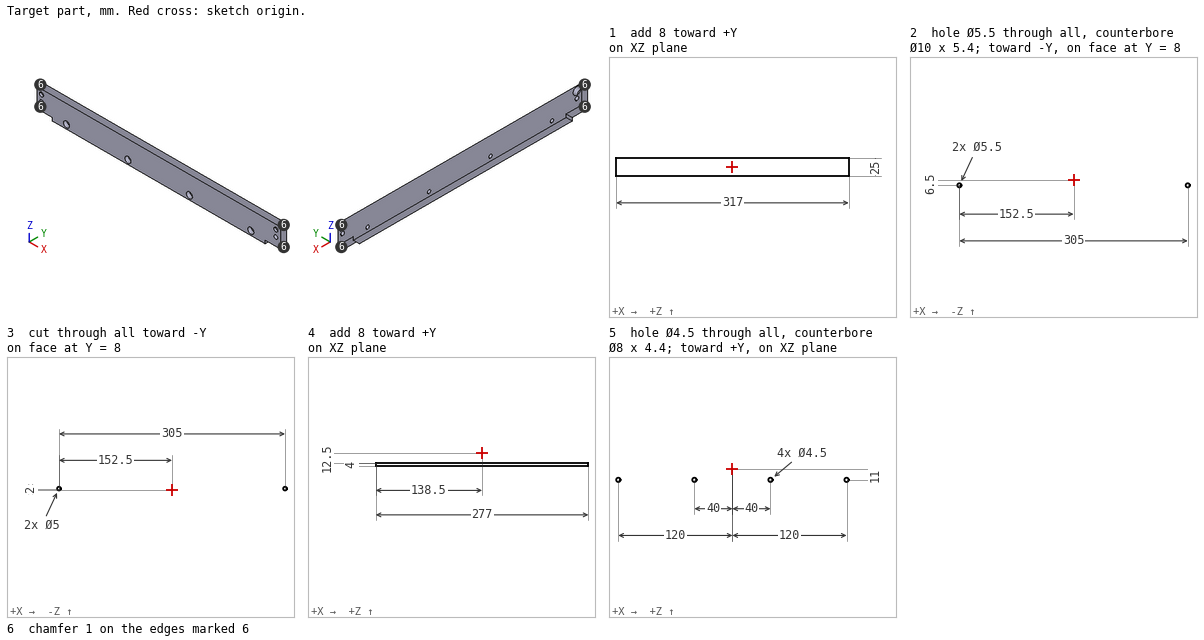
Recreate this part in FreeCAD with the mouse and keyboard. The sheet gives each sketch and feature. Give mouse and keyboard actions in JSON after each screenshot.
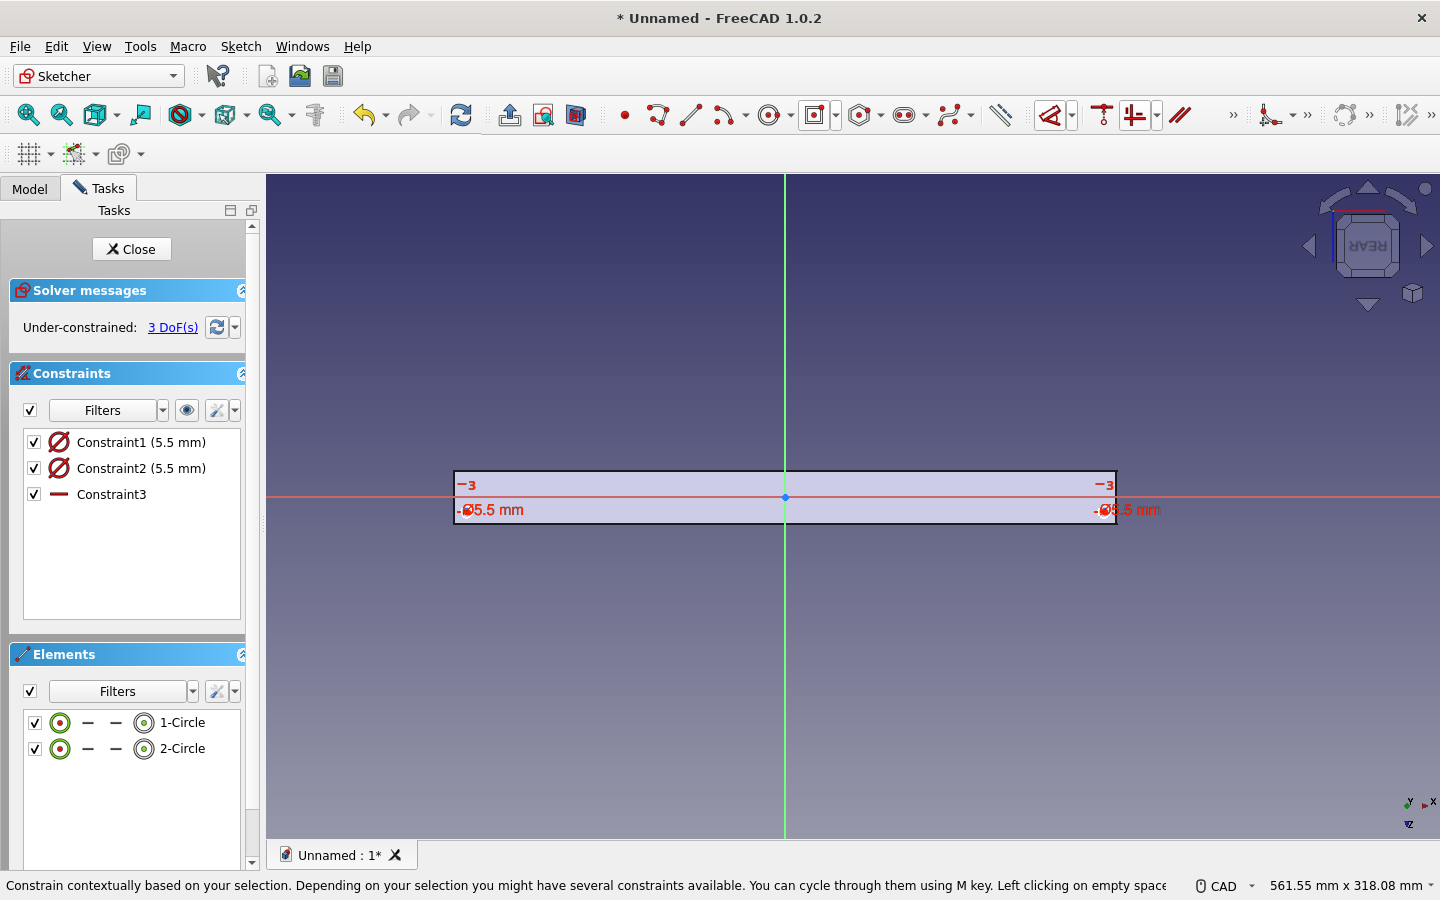
{"action": "scroll", "coordinate": [467, 512], "scroll_direction": "up", "scroll_amount": 6}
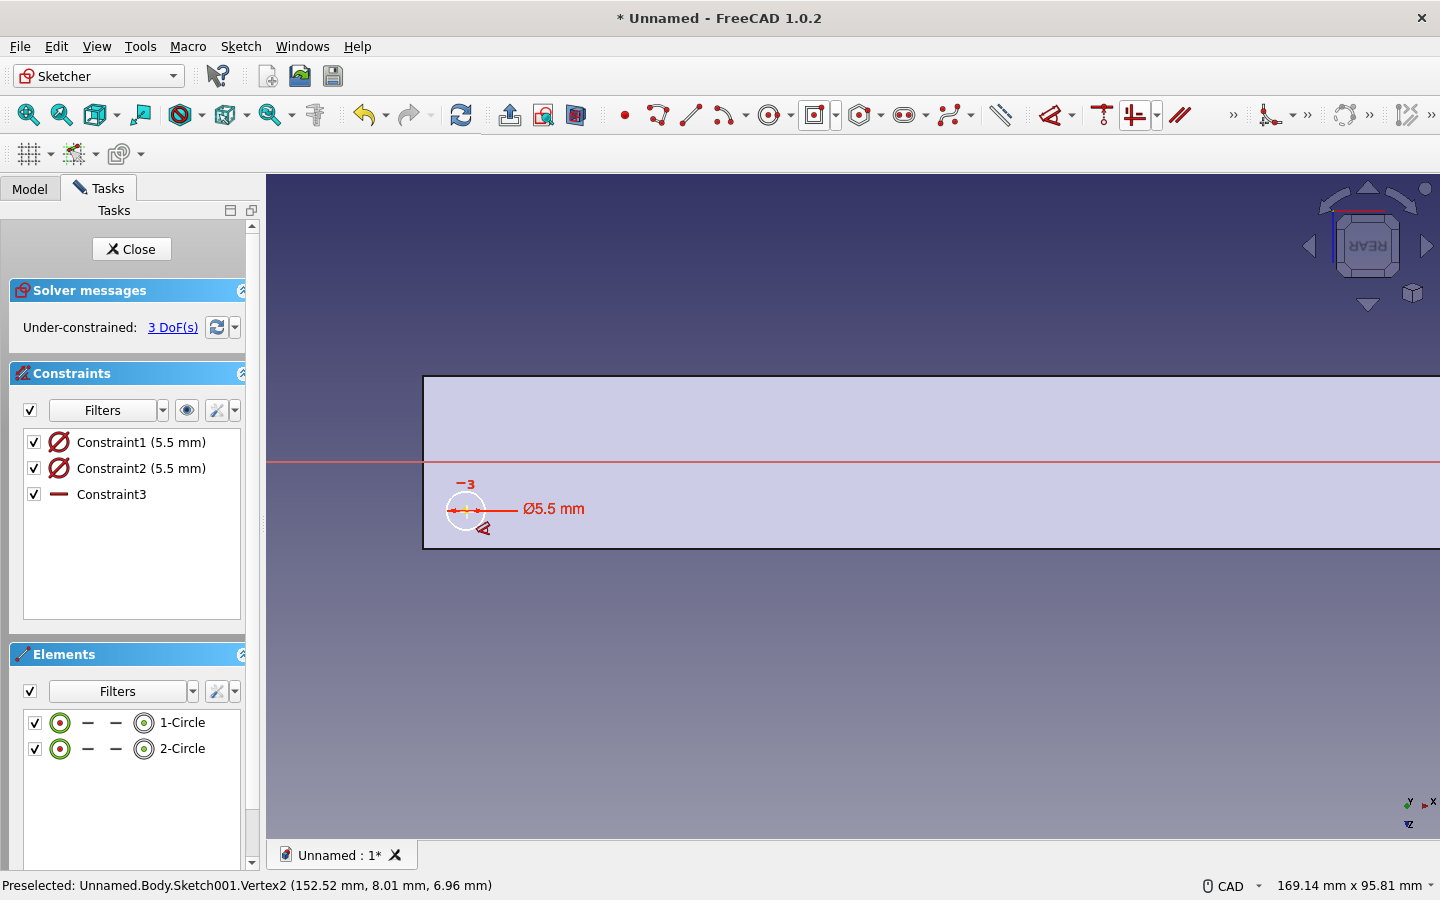
{"action": "left_click", "coordinate": [466, 511]}
{"action": "left_click", "coordinate": [432, 487]}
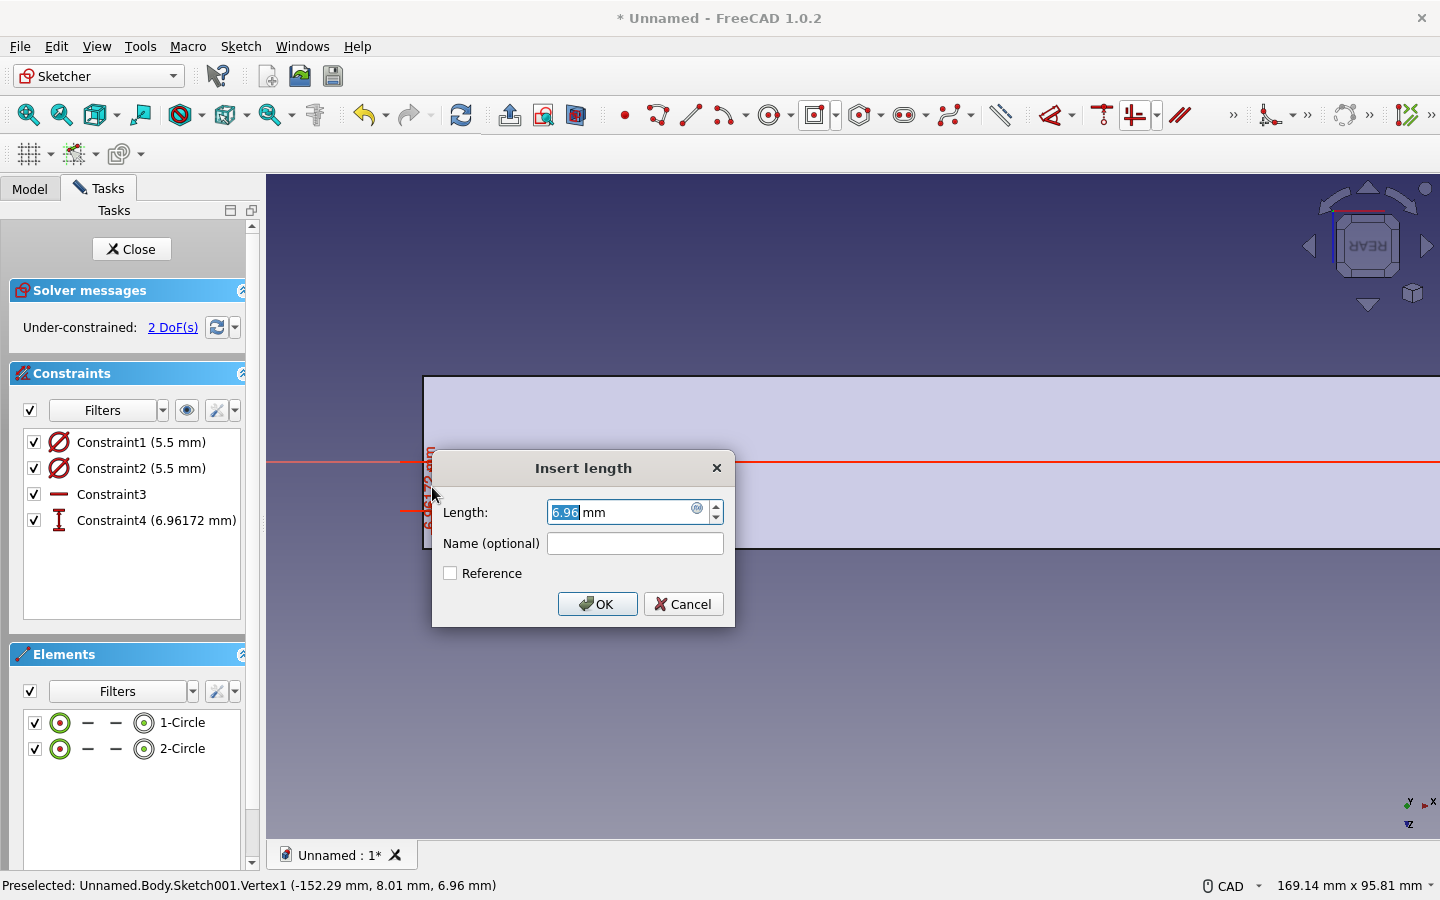
{"action": "type", "text": "6.5"}
{"action": "key", "text": "Return"}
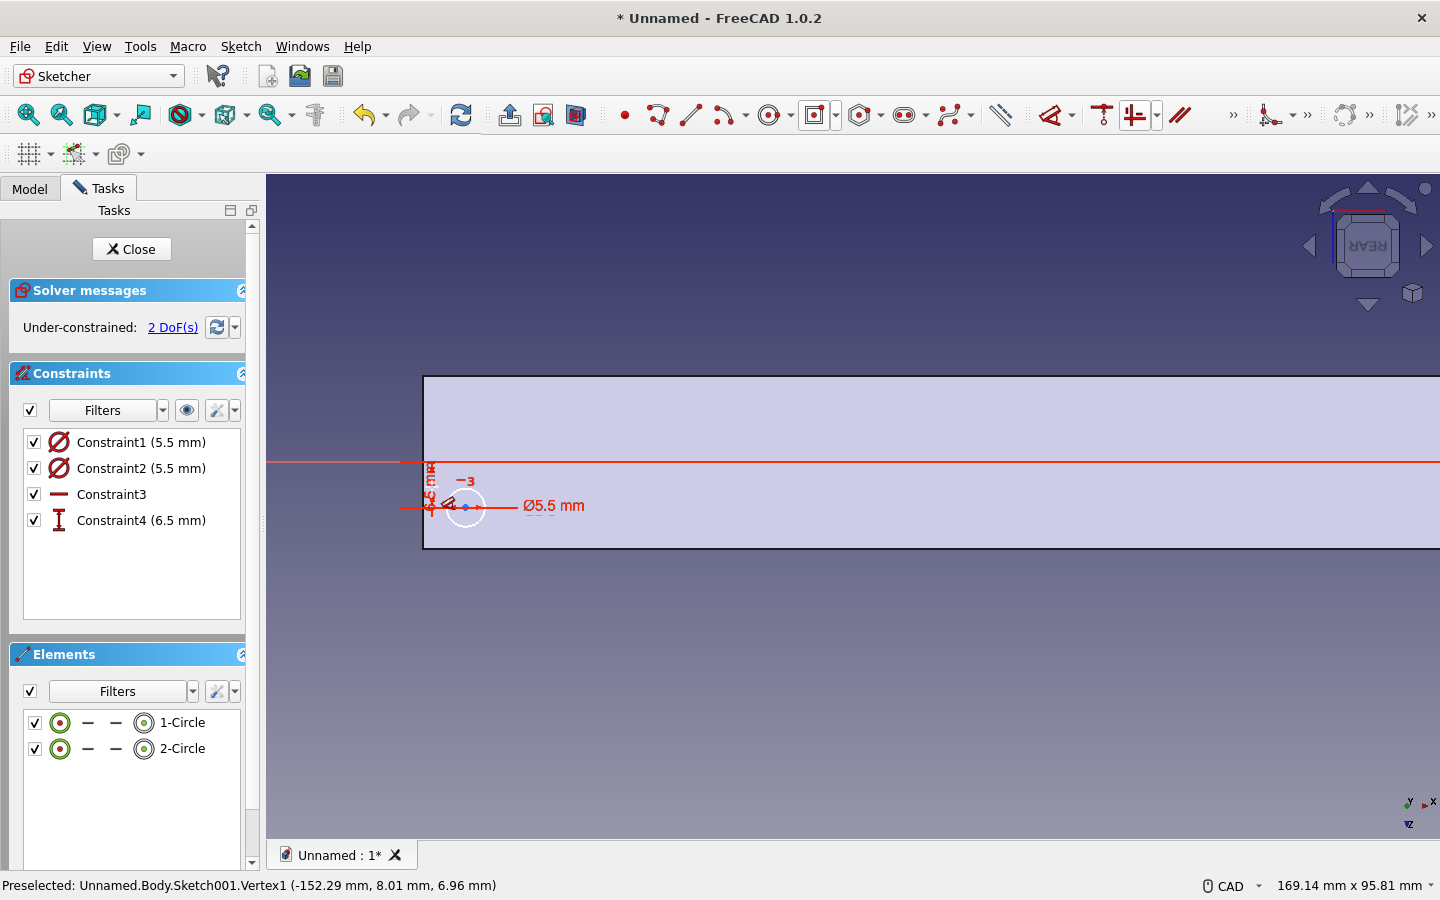
{"action": "left_click", "coordinate": [466, 508]}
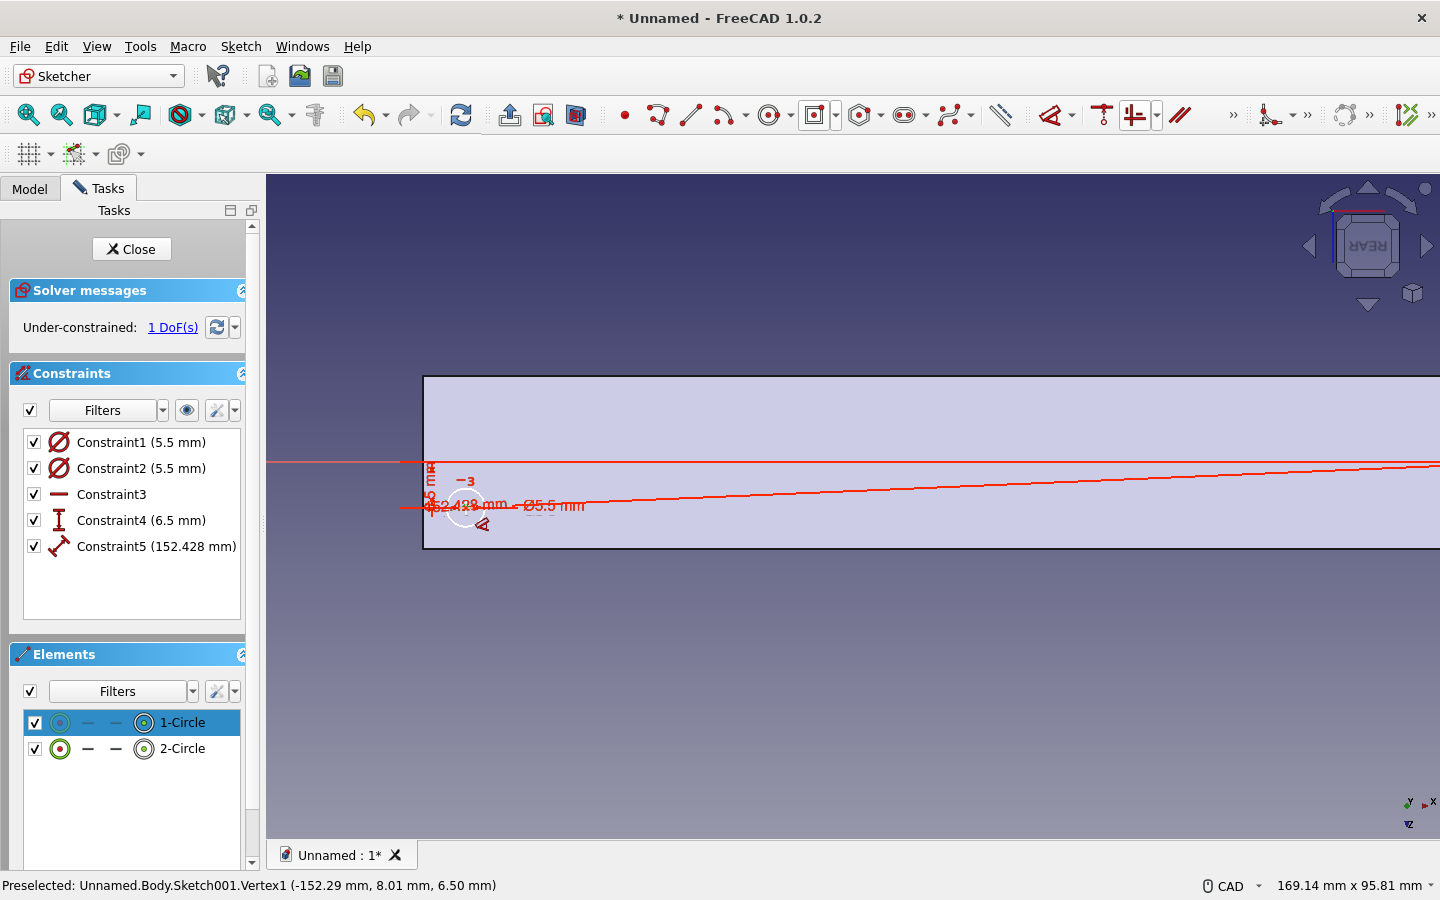
{"action": "scroll", "coordinate": [466, 512], "scroll_direction": "down", "scroll_amount": 6}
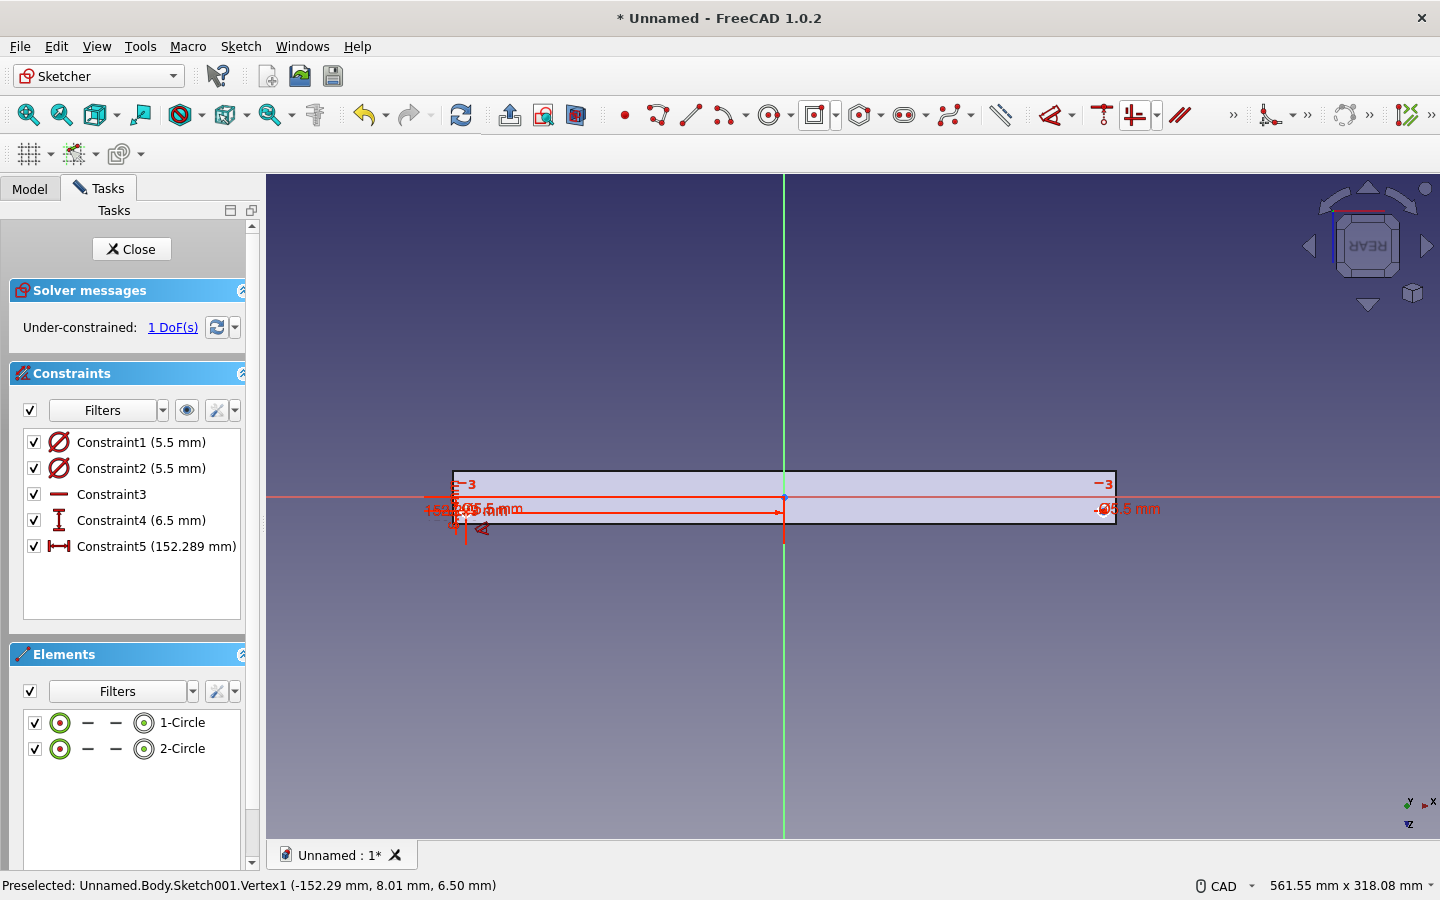
{"action": "left_click", "coordinate": [1103, 511]}
{"action": "left_click", "coordinate": [638, 545]}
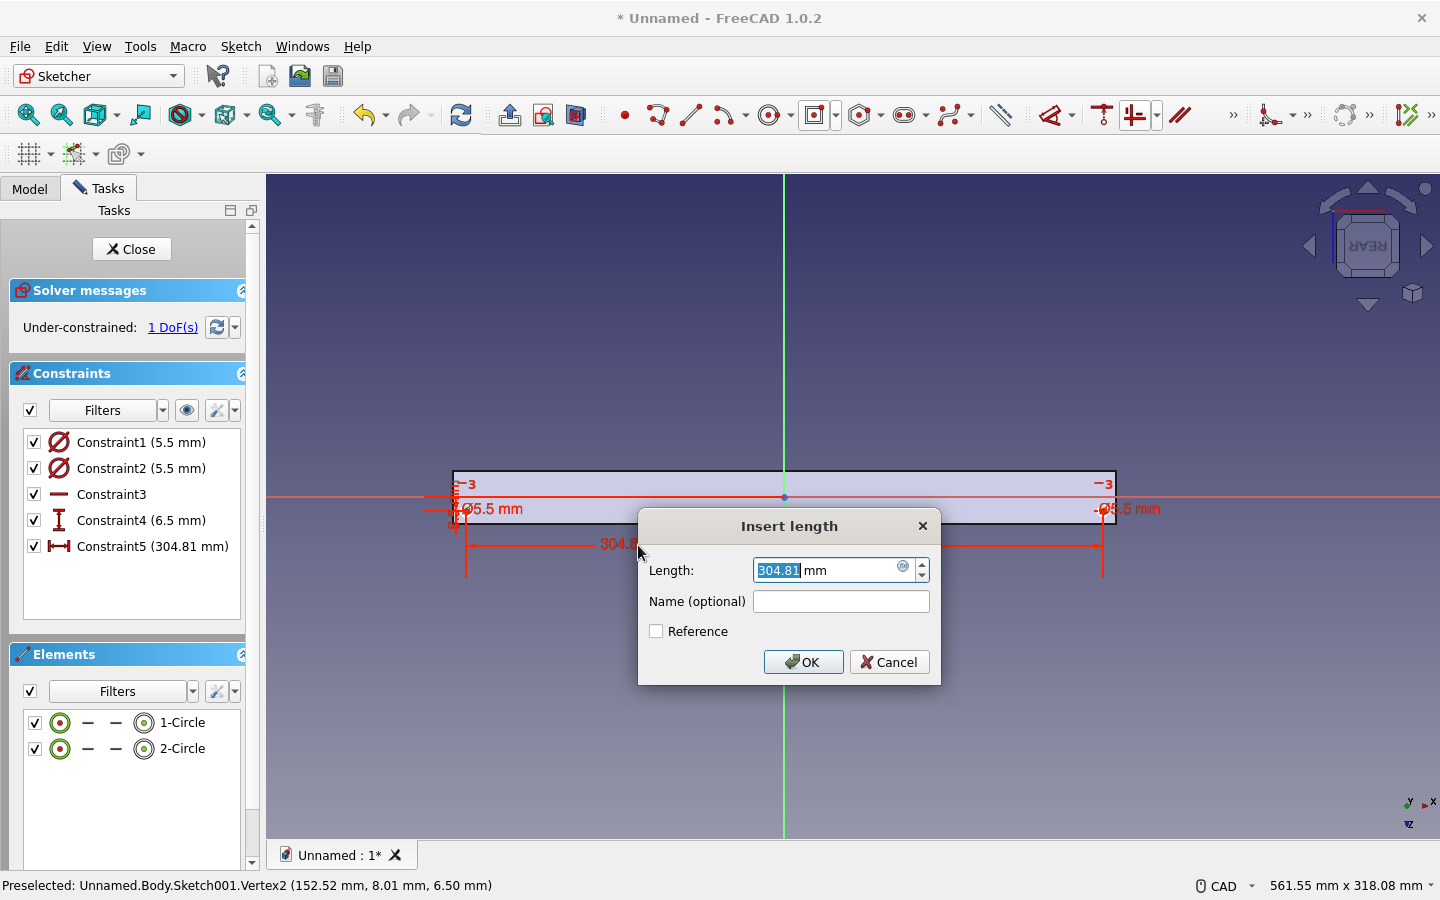
{"action": "type", "text": "305"}
{"action": "key", "text": "Return"}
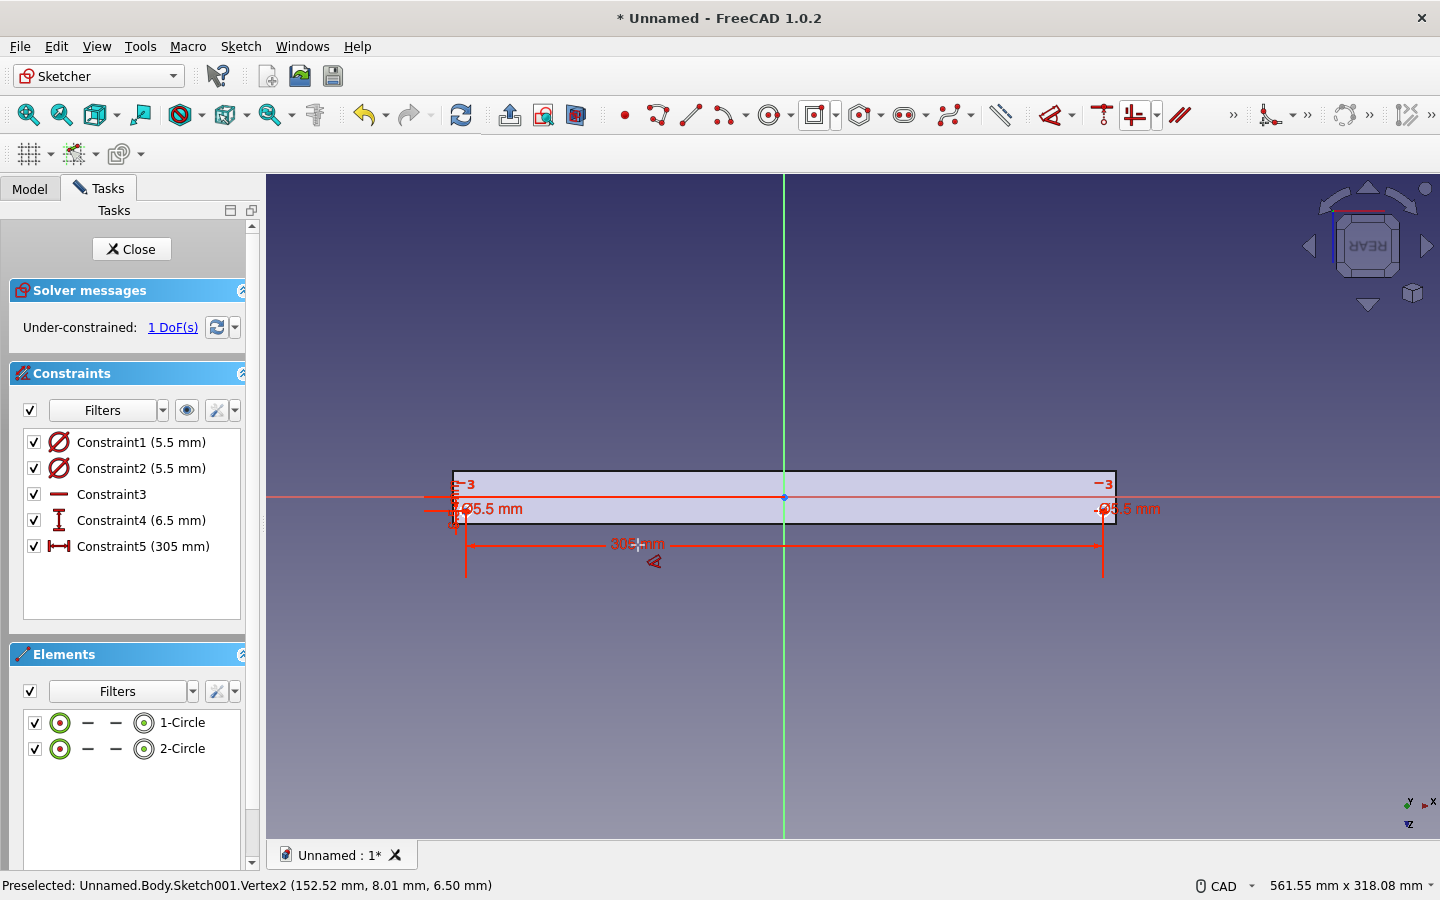
{"action": "left_click", "coordinate": [466, 511]}
{"action": "left_click", "coordinate": [625, 463]}